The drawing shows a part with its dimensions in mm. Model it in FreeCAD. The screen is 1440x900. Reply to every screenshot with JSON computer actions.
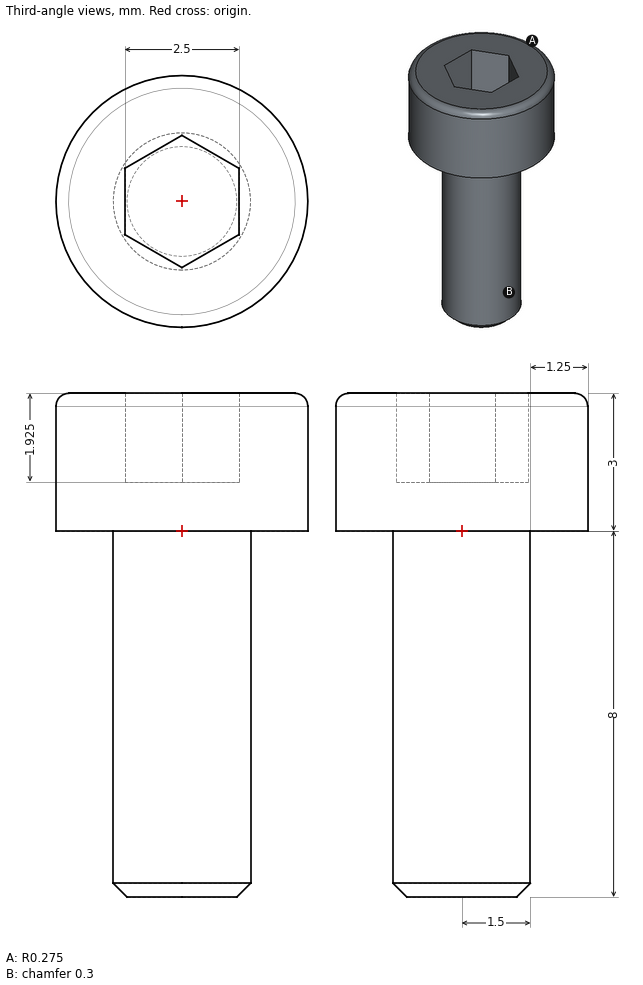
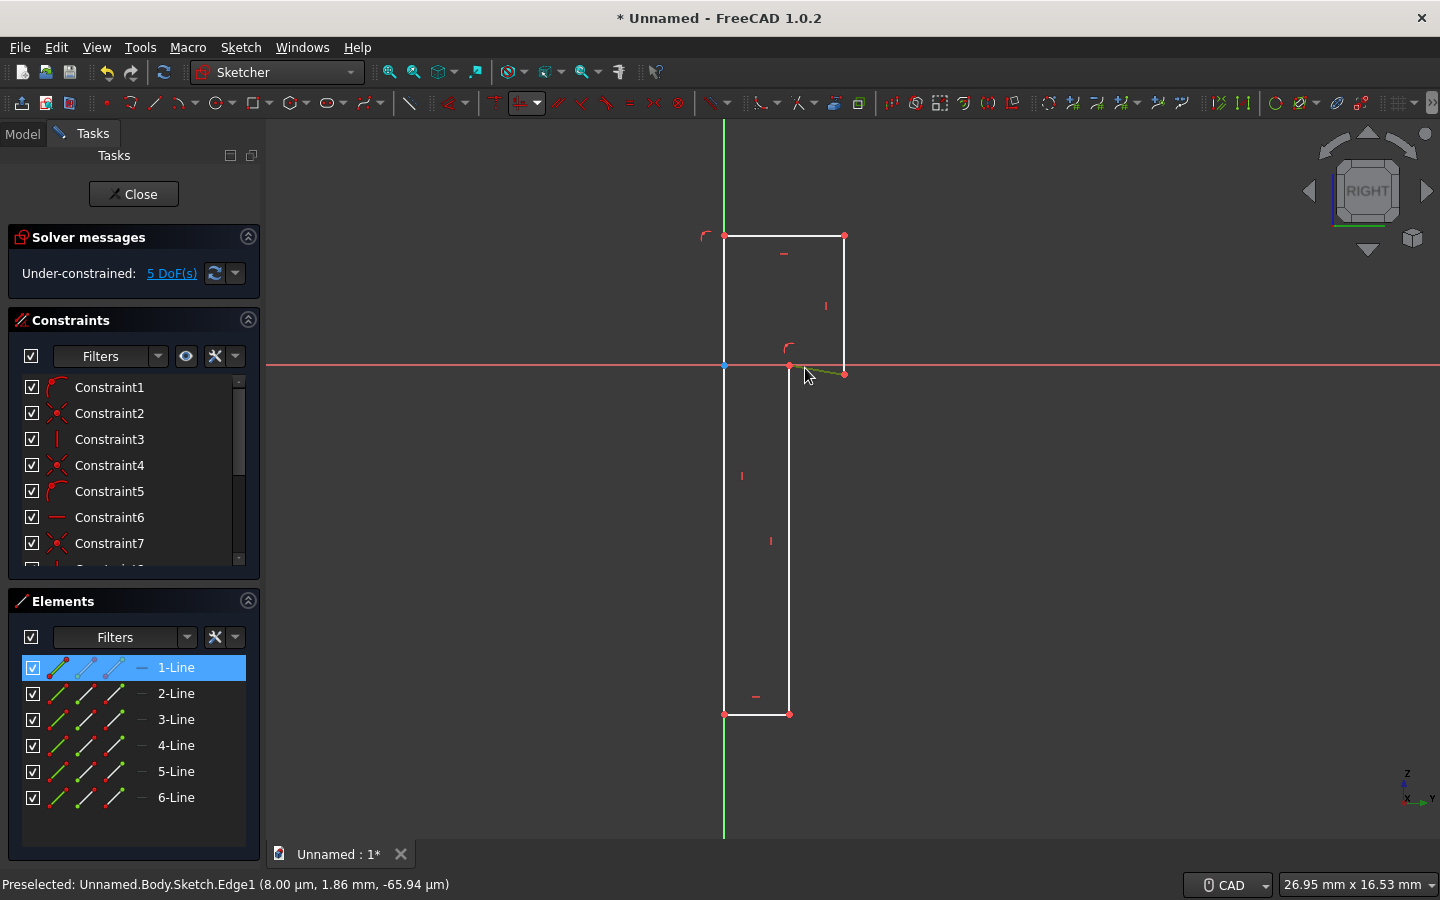
{"action": "key", "text": "h"}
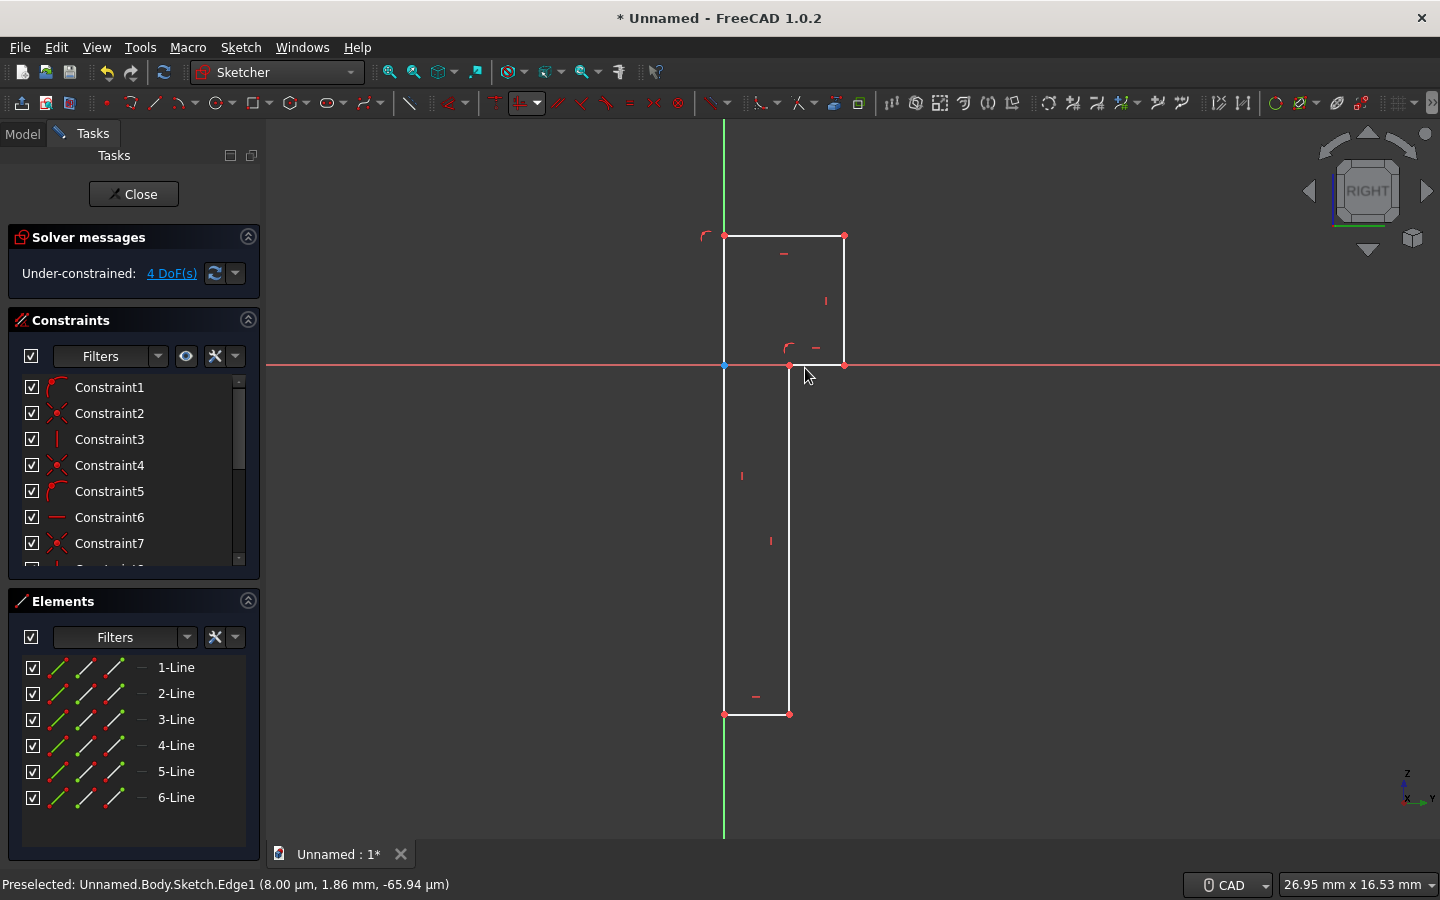
{"action": "left_click", "coordinate": [448, 104]}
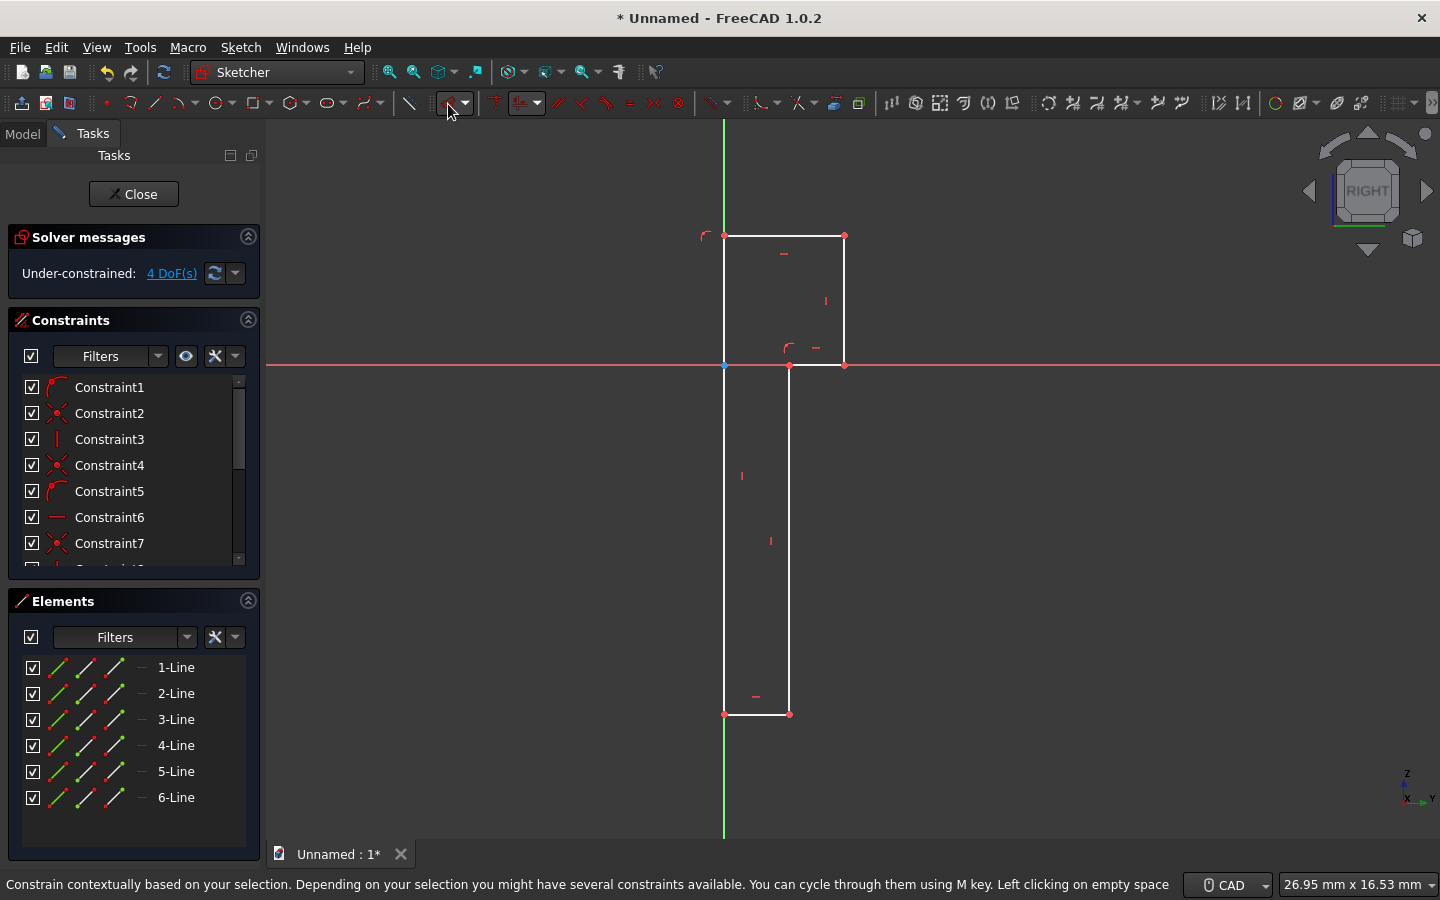
{"action": "left_click", "coordinate": [844, 326]}
{"action": "left_click", "coordinate": [878, 301]}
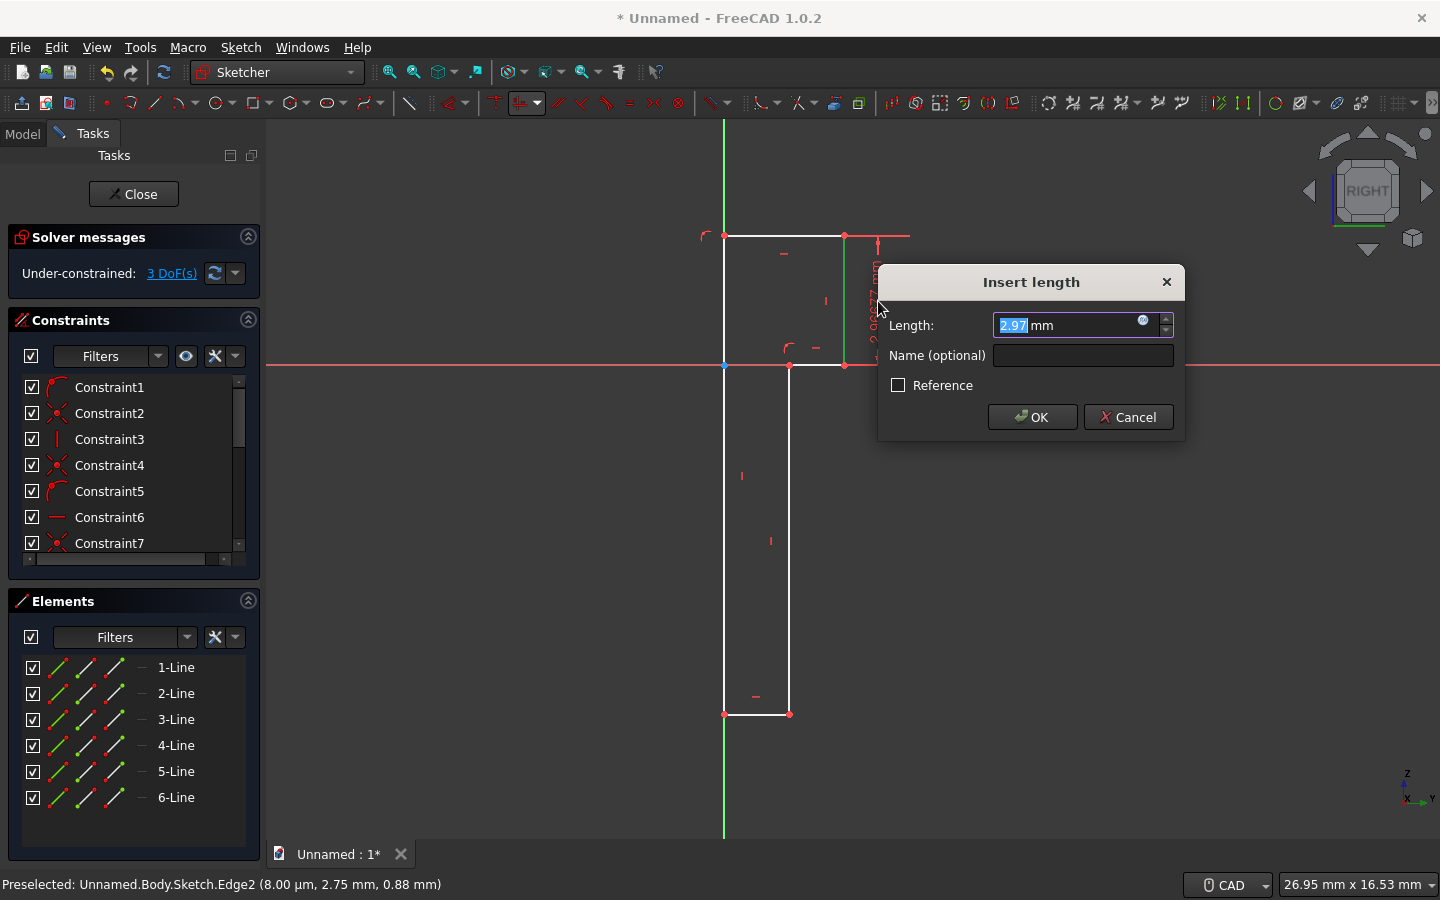
{"action": "type", "text": "3"}
{"action": "key", "text": "Return"}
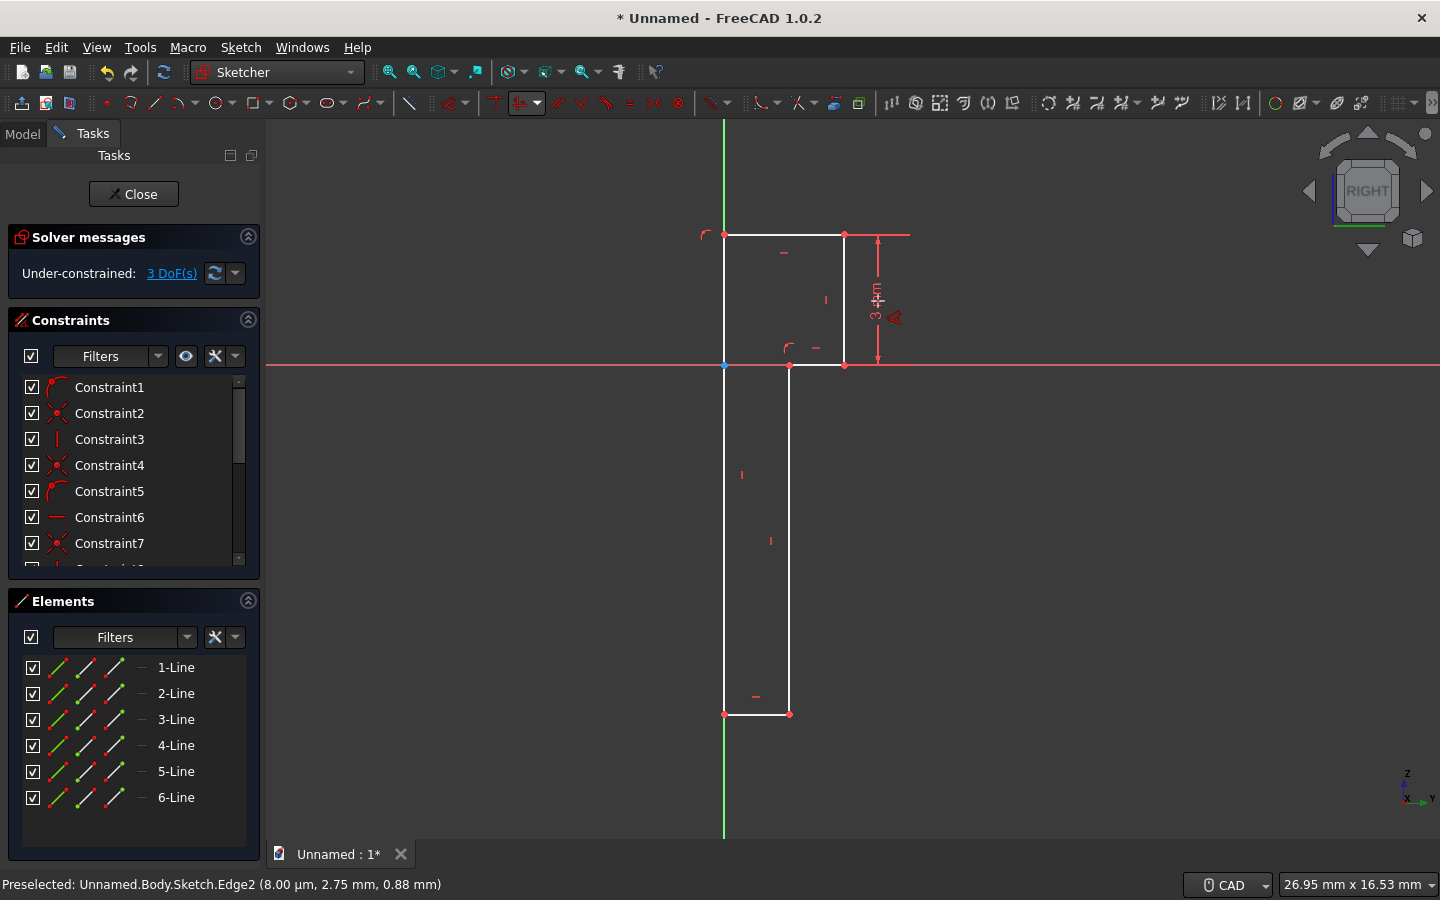
{"action": "left_click", "coordinate": [789, 610]}
{"action": "left_click", "coordinate": [823, 540]}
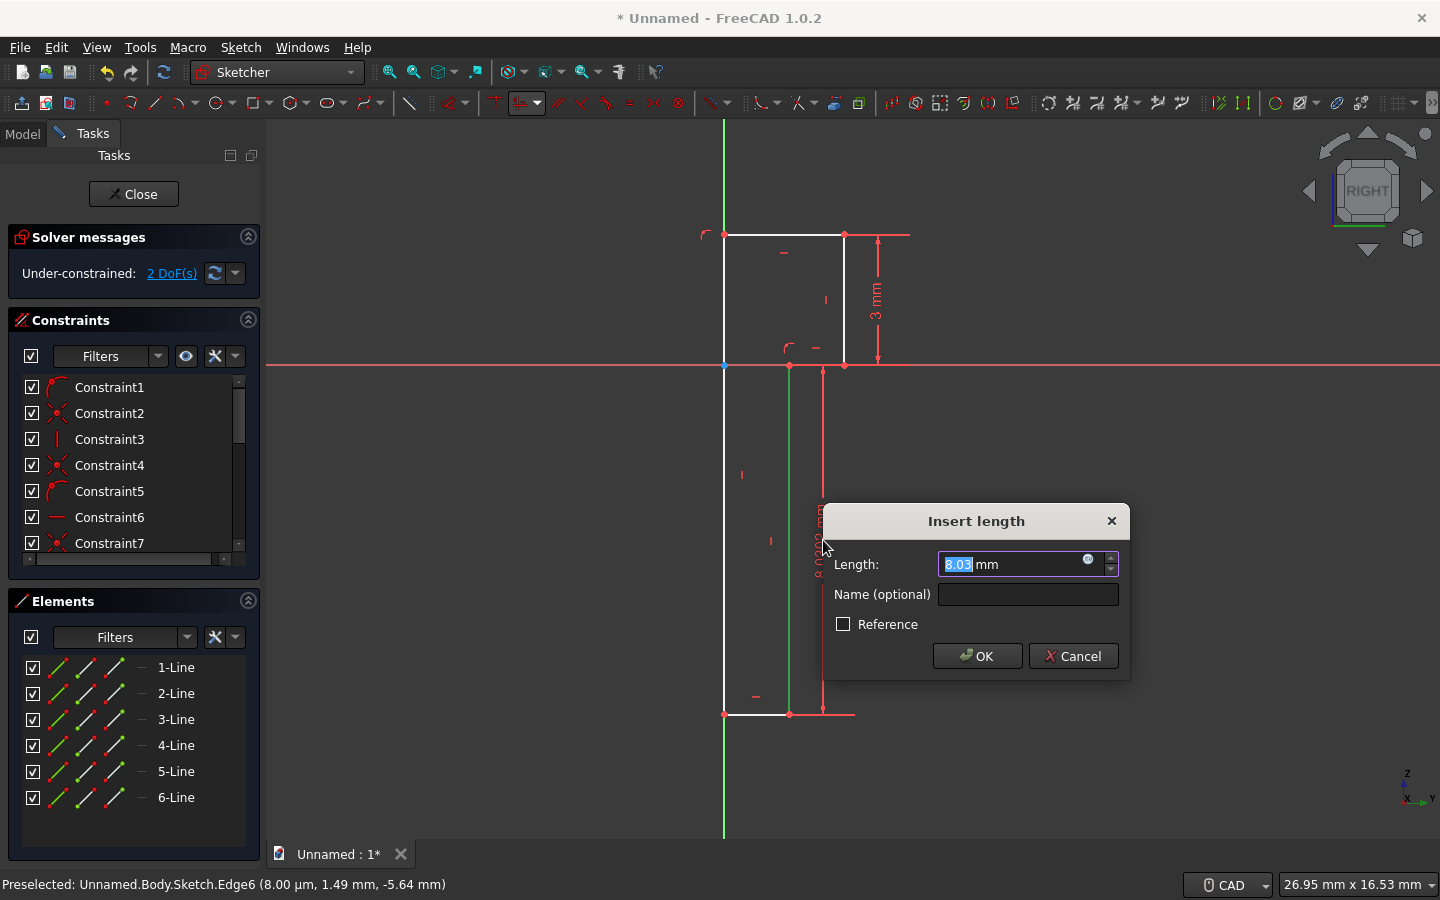
{"action": "type", "text": "8"}
{"action": "key", "text": "Return"}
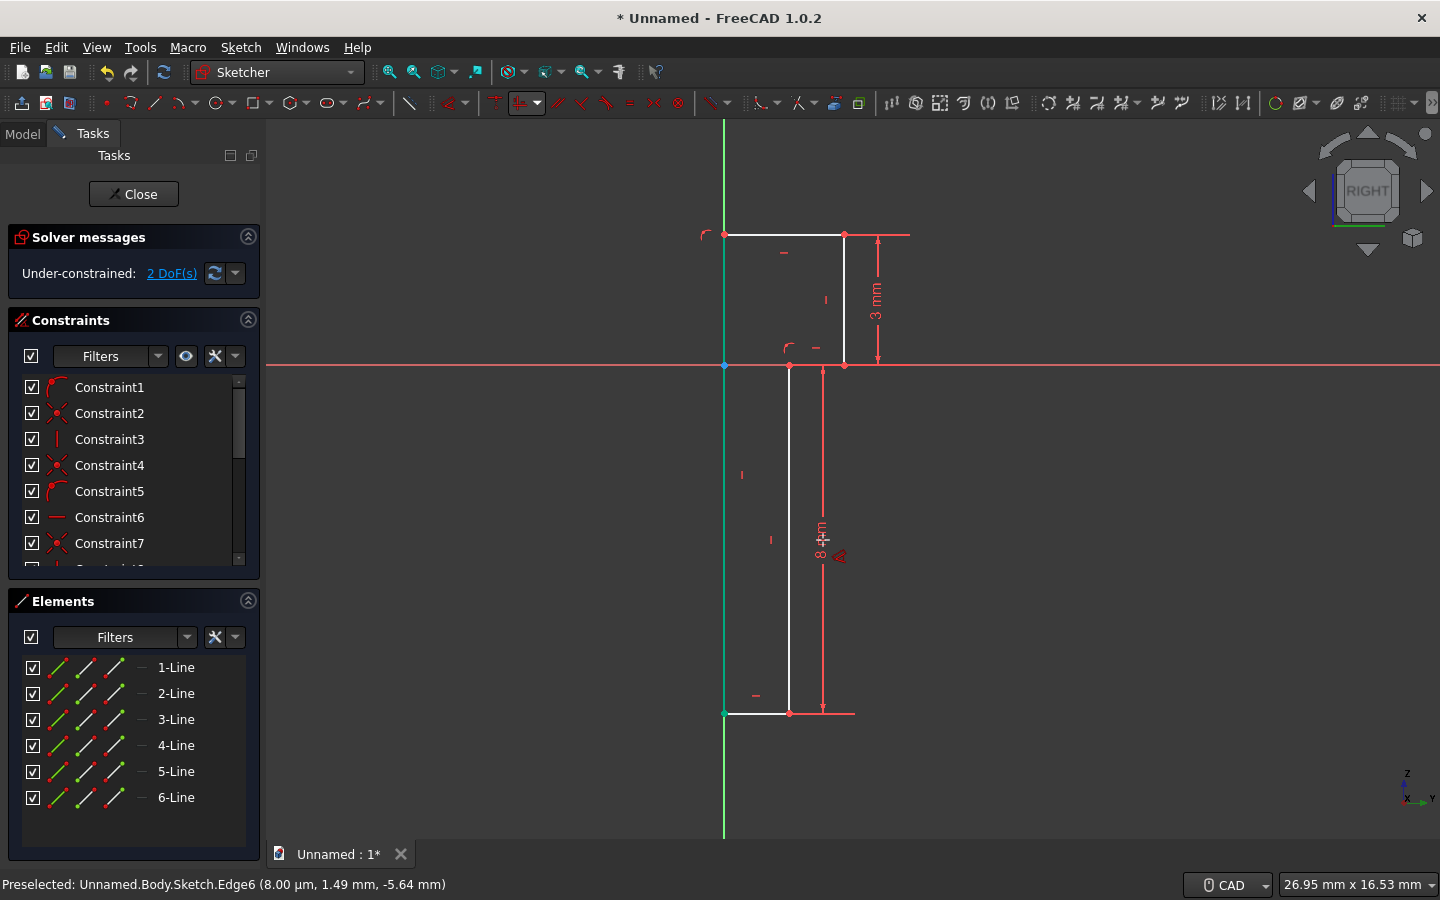
{"action": "left_click", "coordinate": [744, 714]}
{"action": "left_click", "coordinate": [757, 748]}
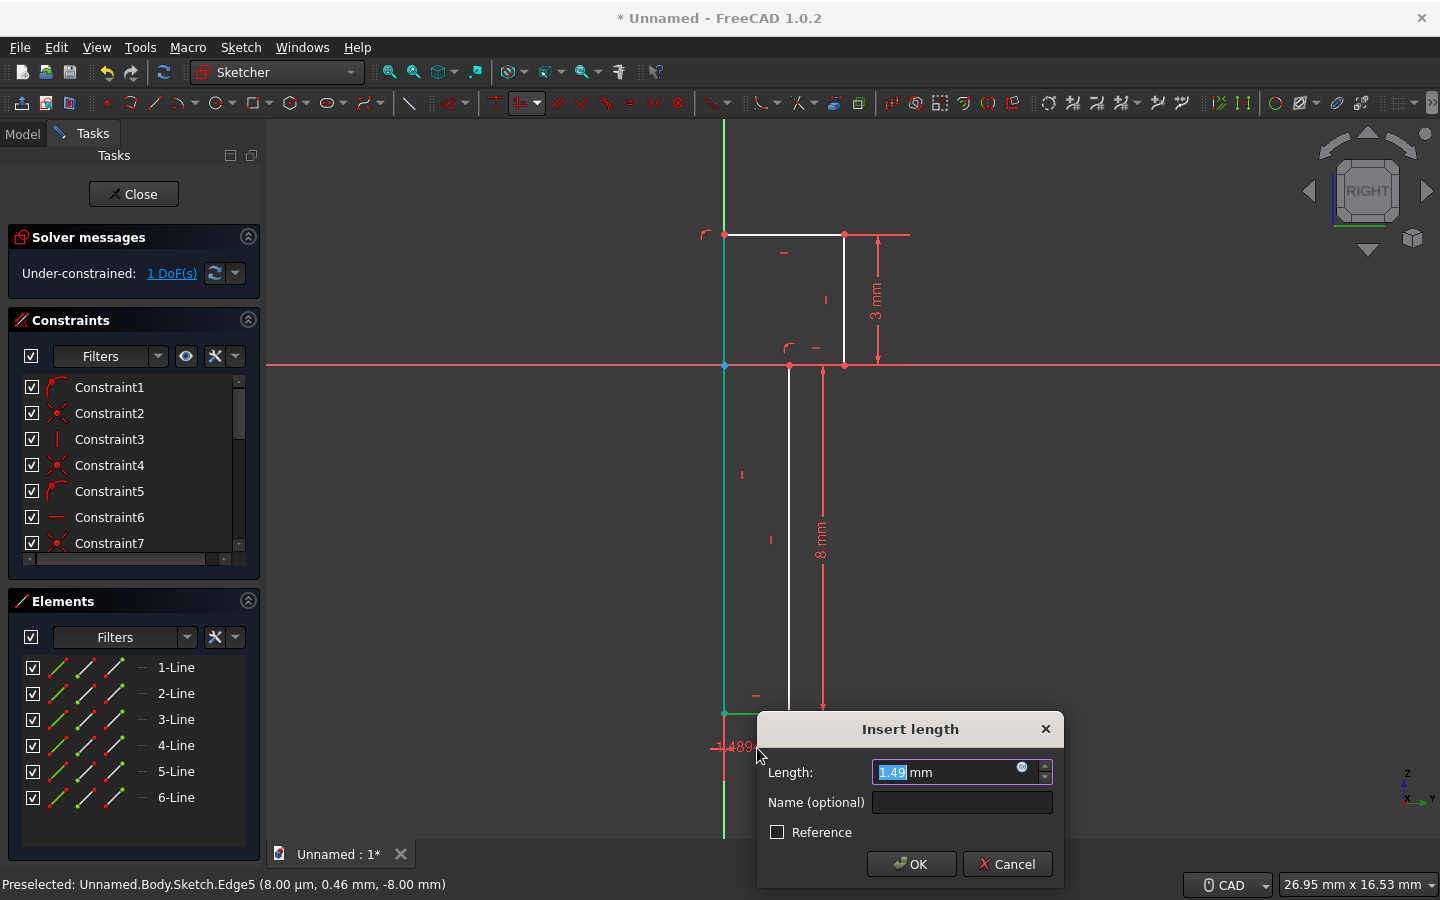
{"action": "type", "text": "1.5"}
{"action": "key", "text": "Return"}